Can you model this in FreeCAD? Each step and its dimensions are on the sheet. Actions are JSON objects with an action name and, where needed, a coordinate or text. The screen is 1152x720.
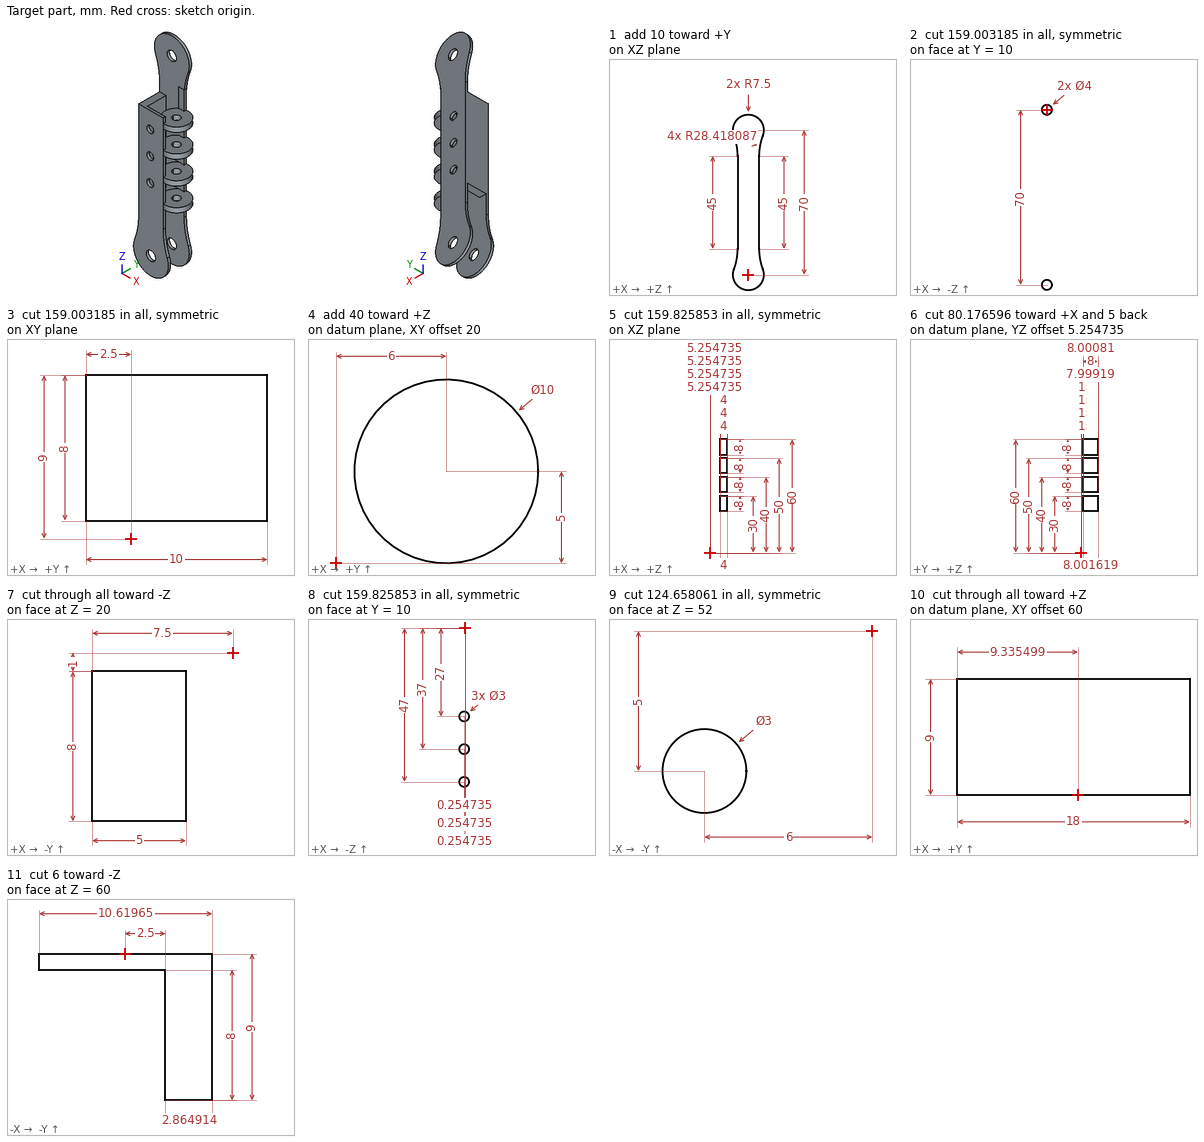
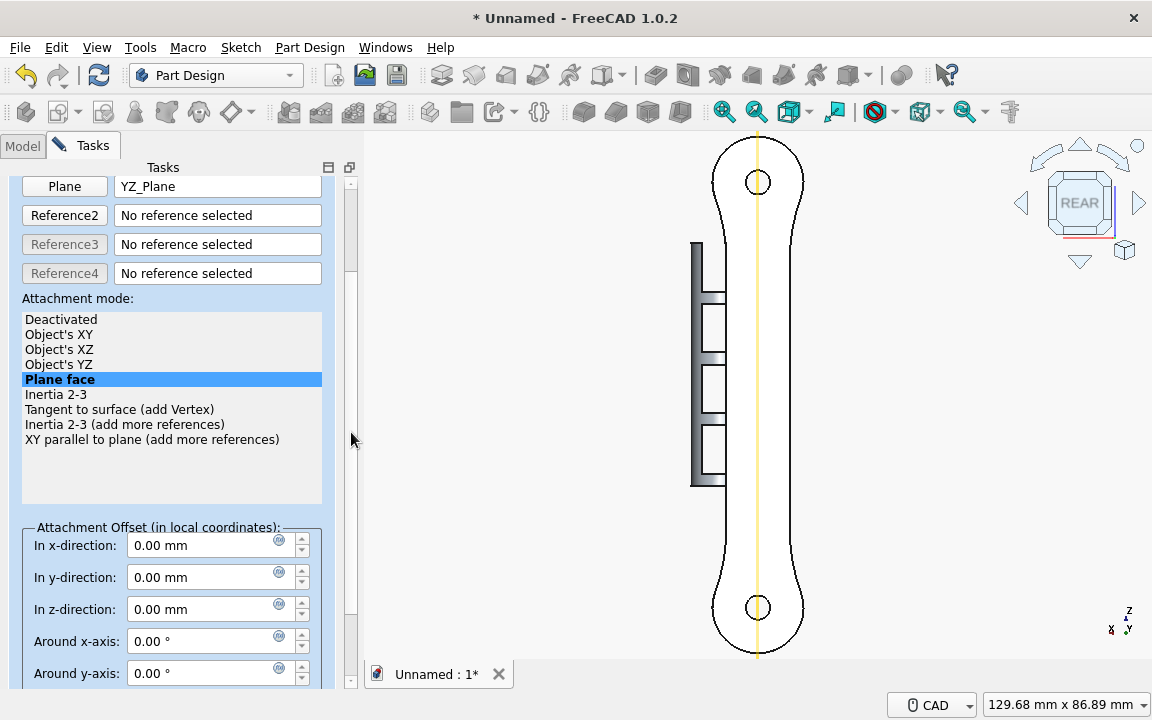
{"action": "triple_click", "coordinate": [210, 609]}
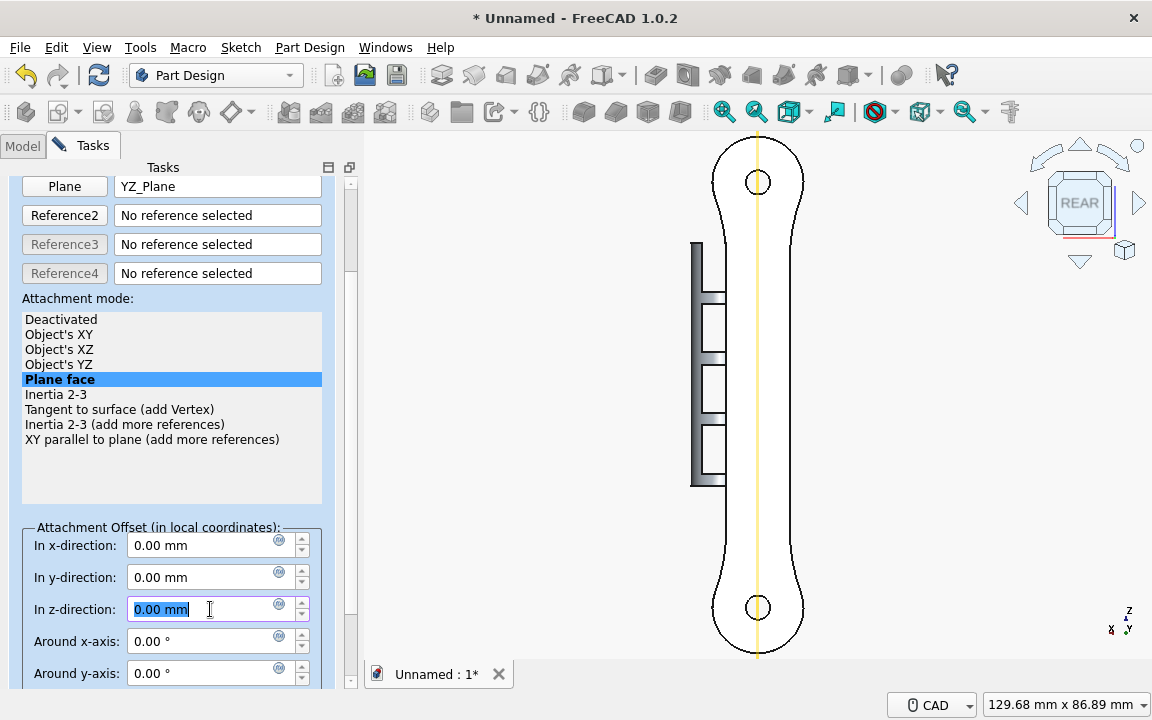
{"action": "type", "text": "5.254735"}
{"action": "key", "text": "Tab"}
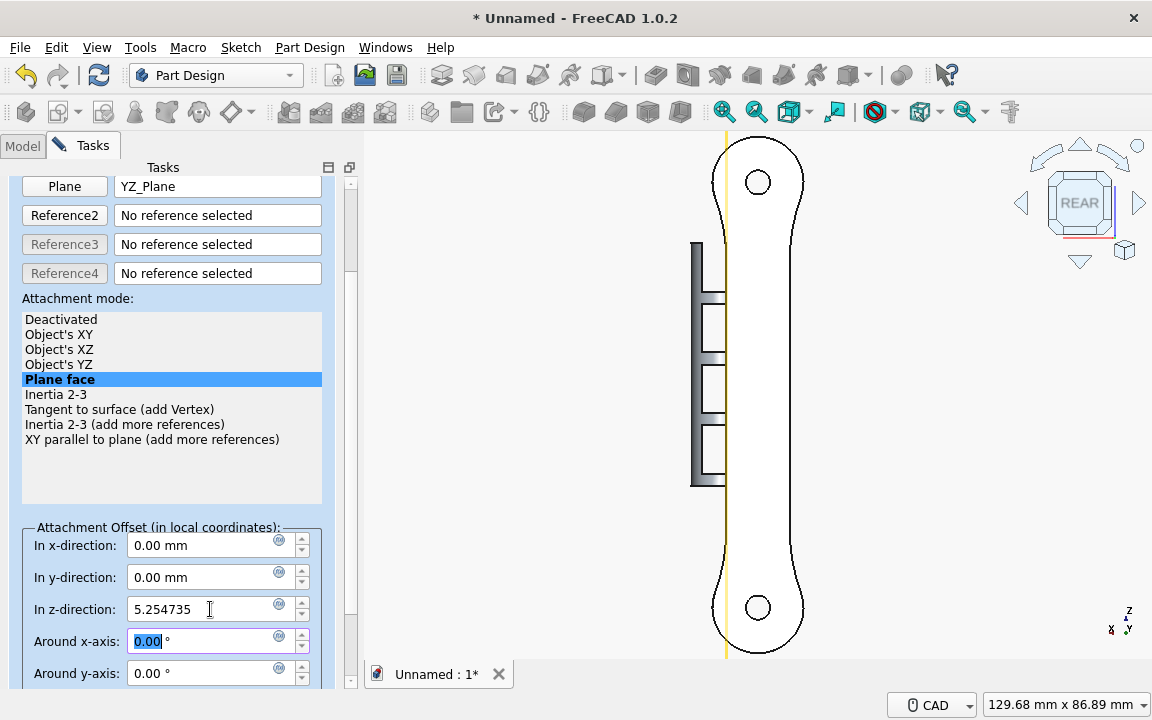
{"action": "scroll", "coordinate": [351, 432], "scroll_direction": "up", "scroll_amount": 3}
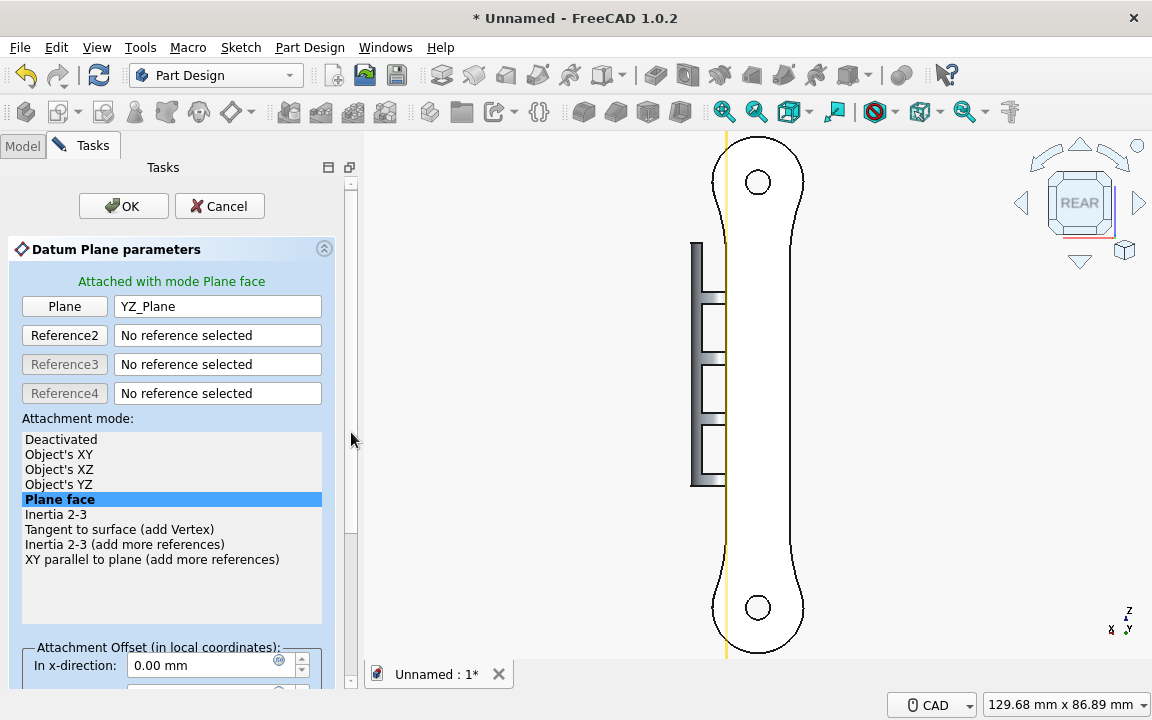
{"action": "left_click", "coordinate": [124, 206]}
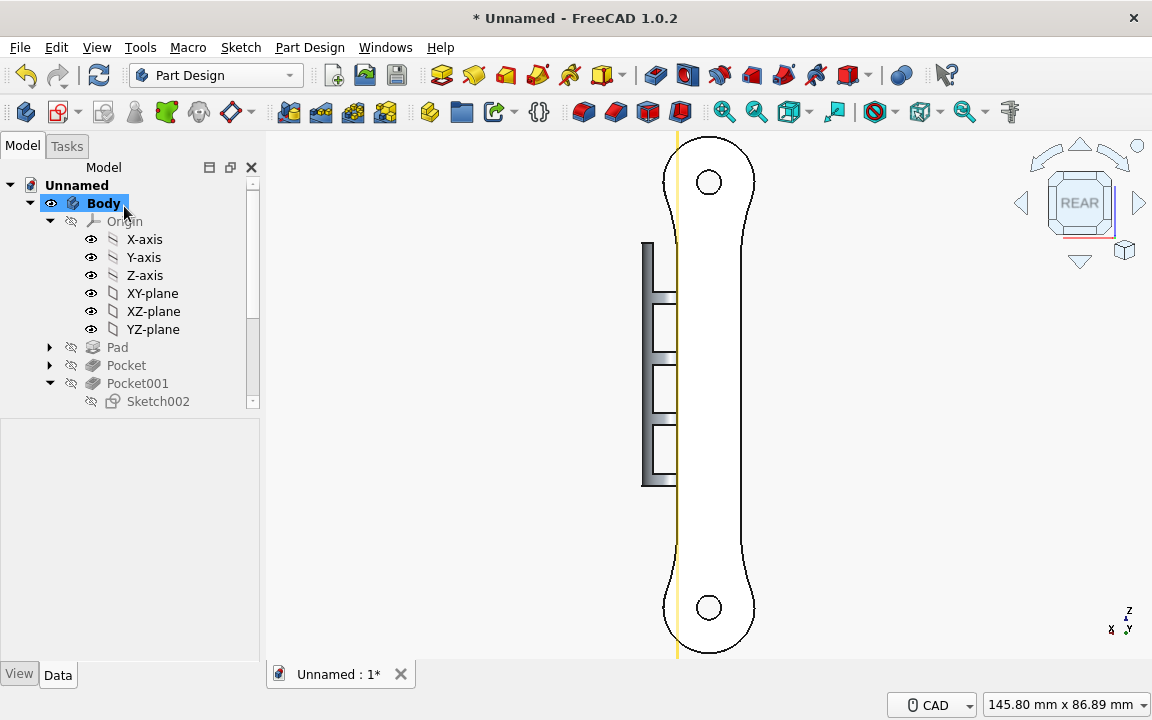
{"action": "scroll", "coordinate": [100, 289], "scroll_direction": "down", "scroll_amount": 3}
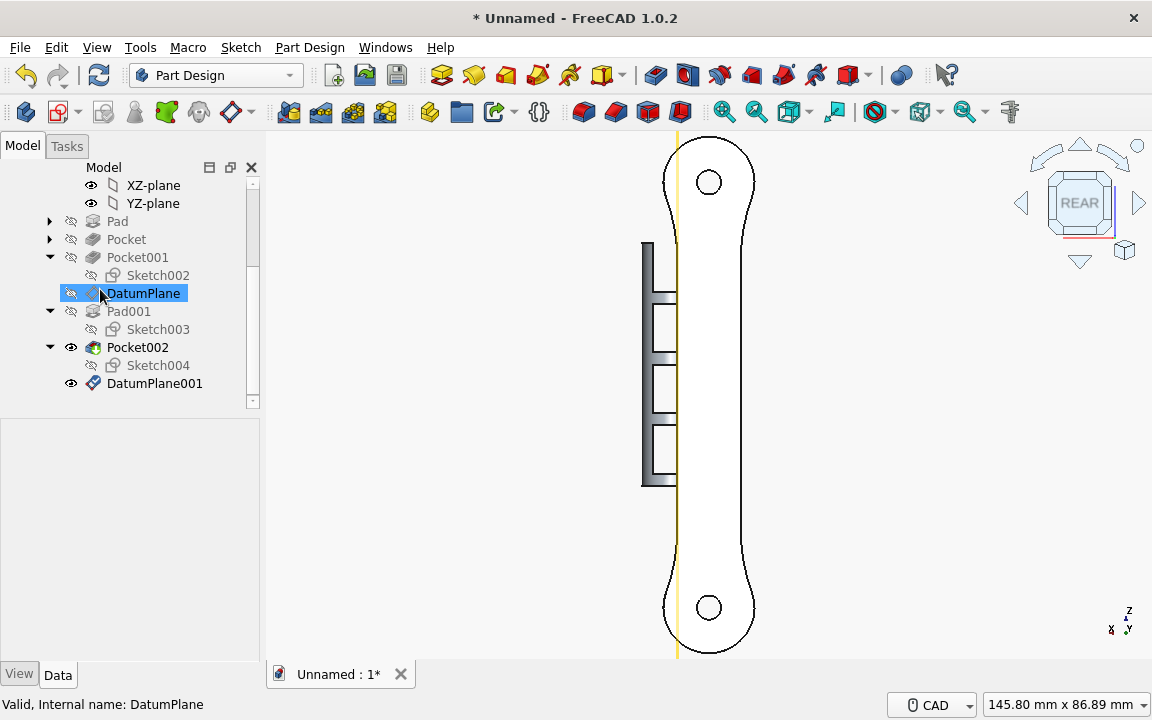
{"action": "left_click", "coordinate": [116, 383]}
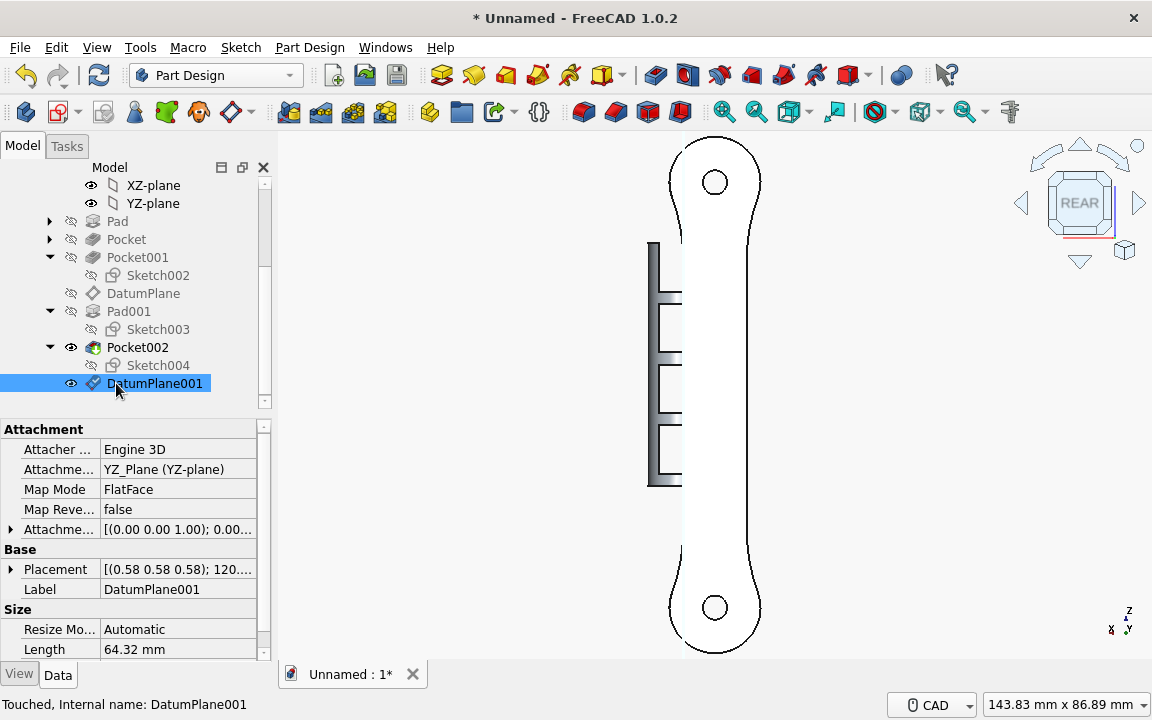
{"action": "left_click", "coordinate": [58, 112]}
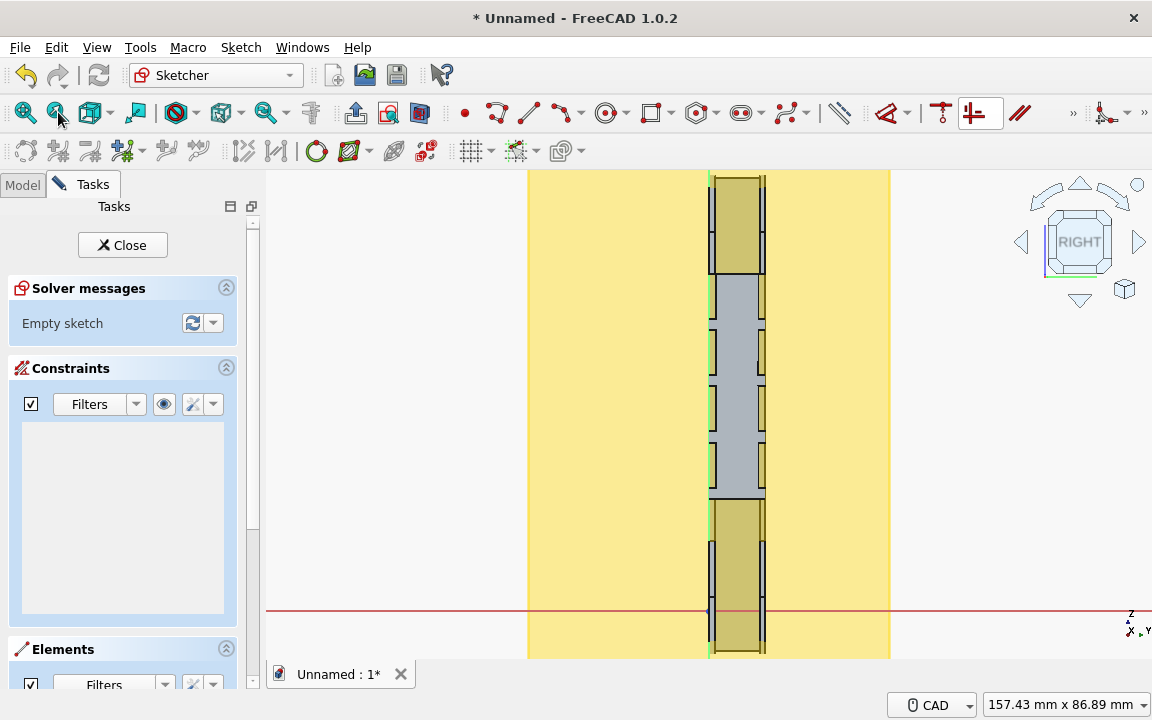
{"action": "left_click", "coordinate": [420, 114]}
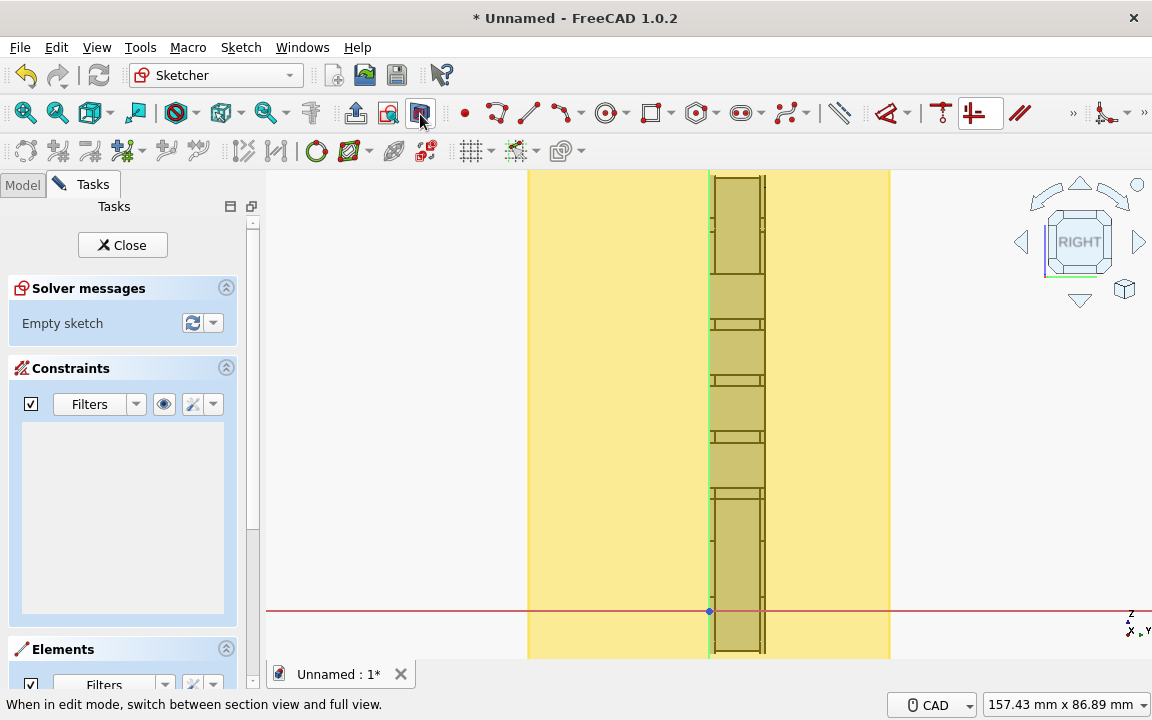
{"action": "scroll", "coordinate": [294, 287], "scroll_direction": "down", "scroll_amount": 1}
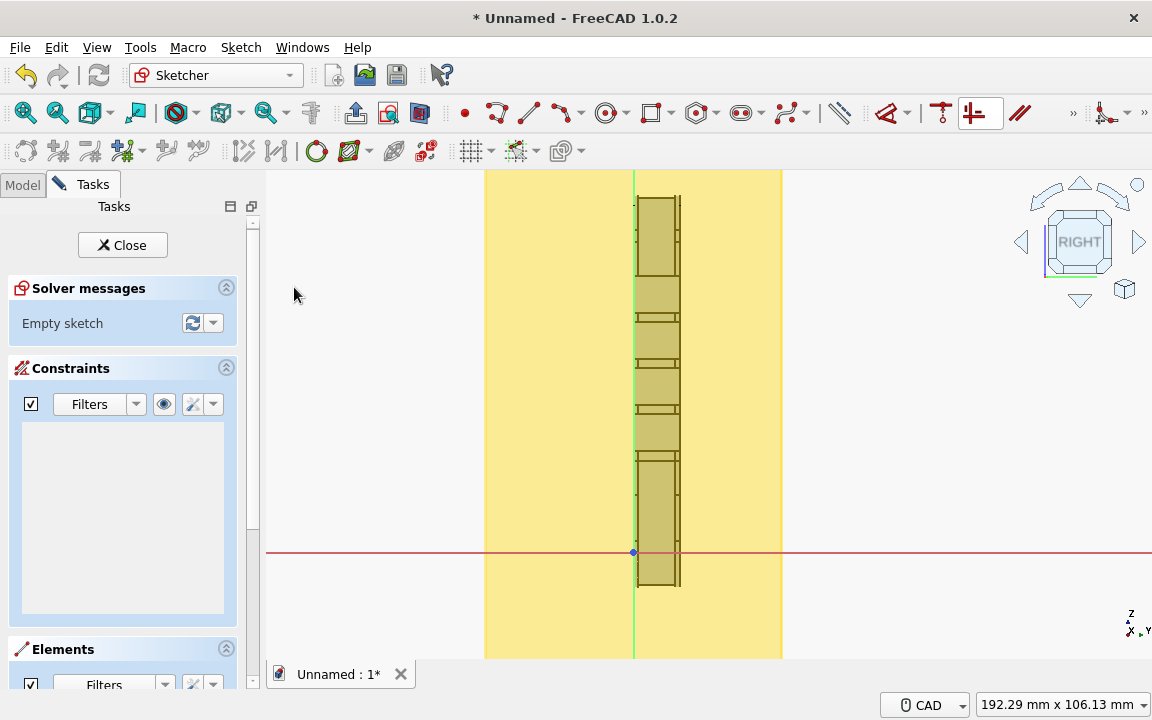
{"action": "key", "text": "g r"}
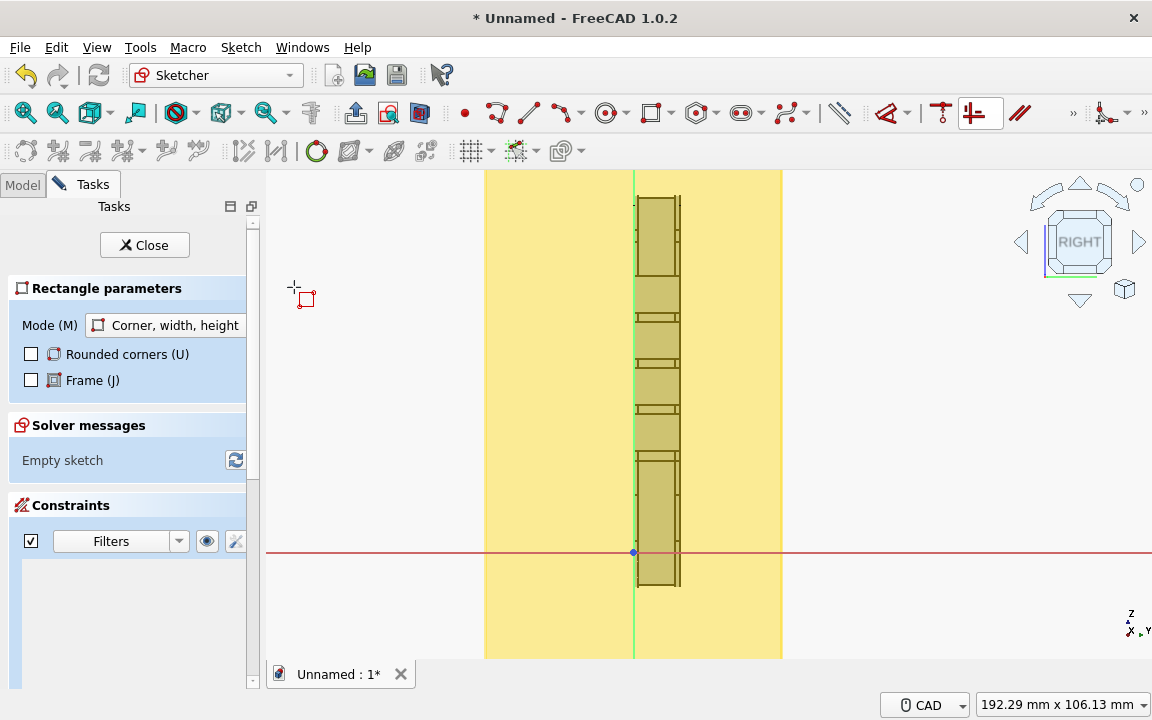
{"action": "scroll", "coordinate": [638, 276], "scroll_direction": "up", "scroll_amount": 7}